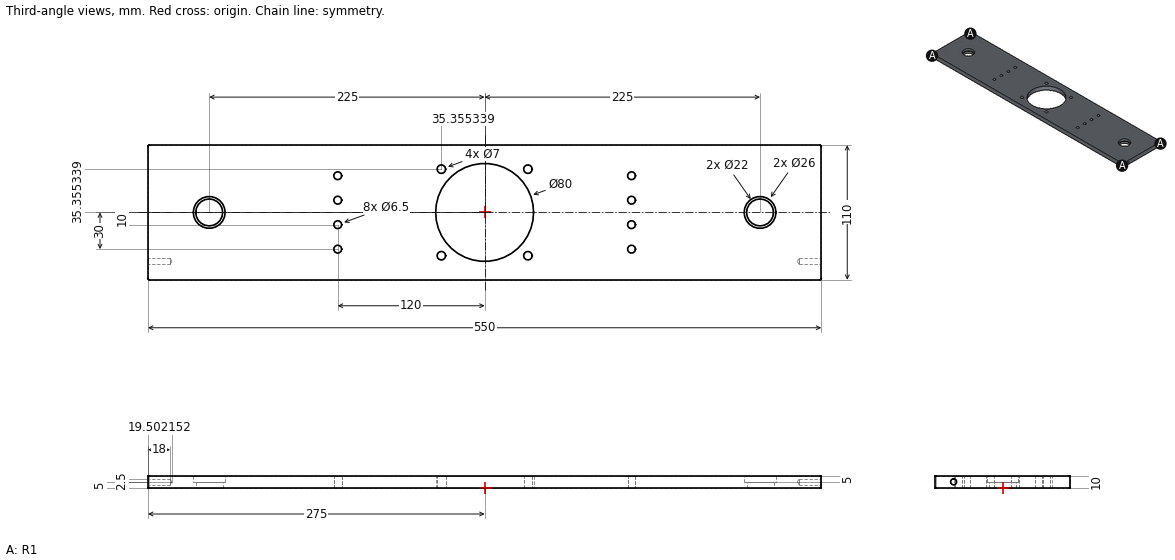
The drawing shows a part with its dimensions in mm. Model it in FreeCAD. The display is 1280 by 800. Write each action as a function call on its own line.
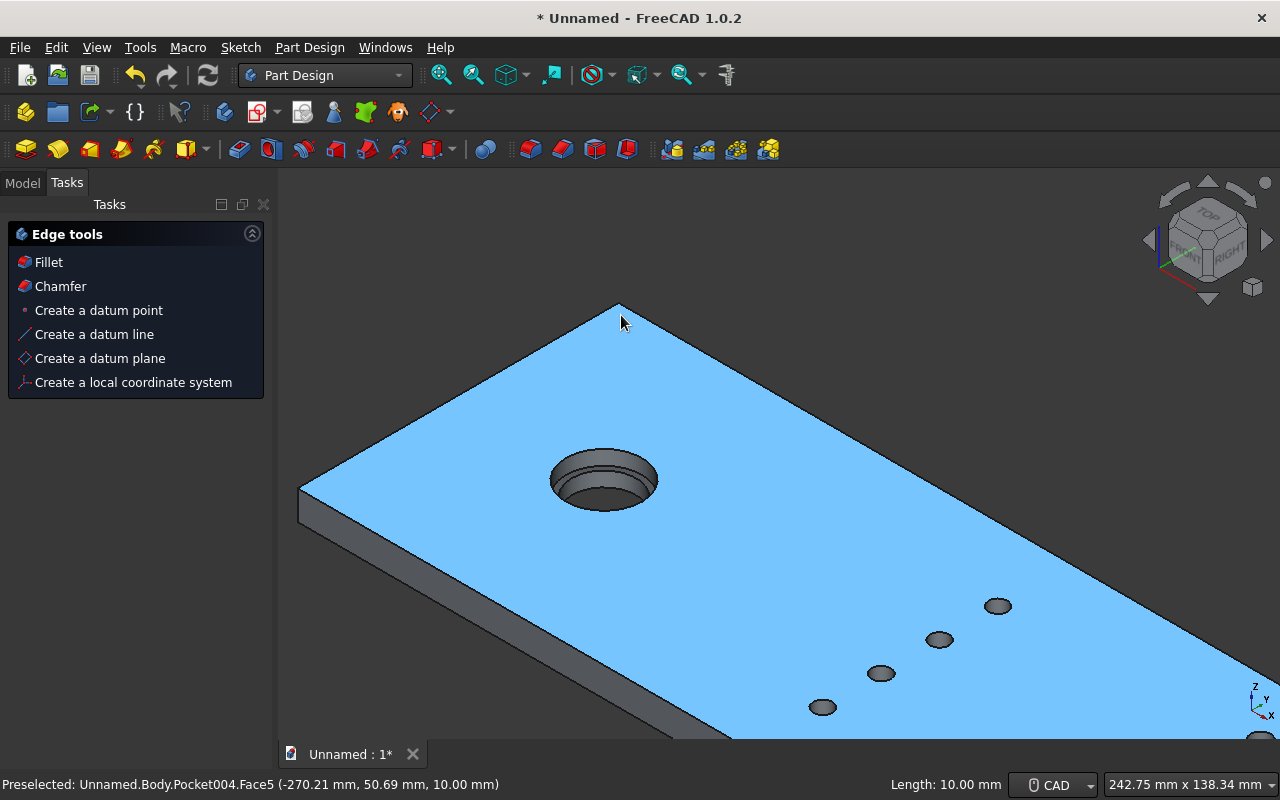
key(v)
key(f)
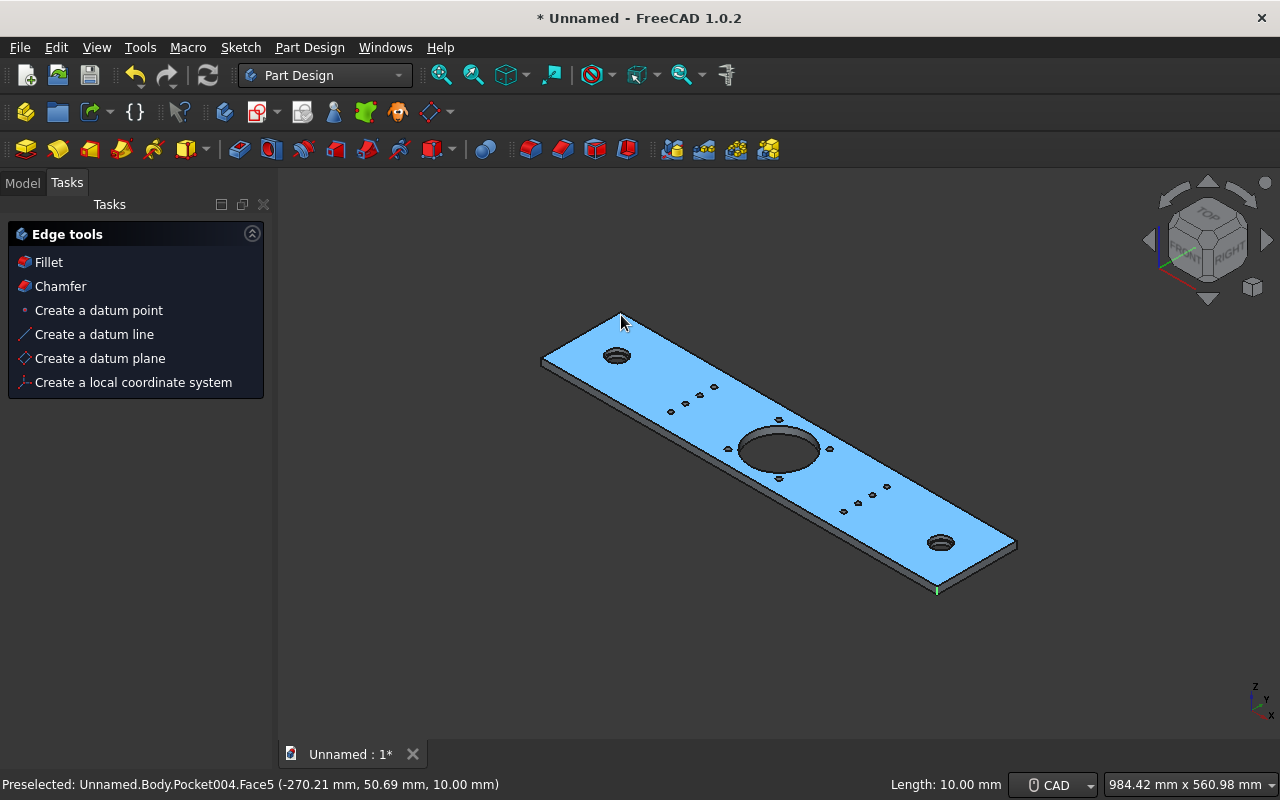
key(2)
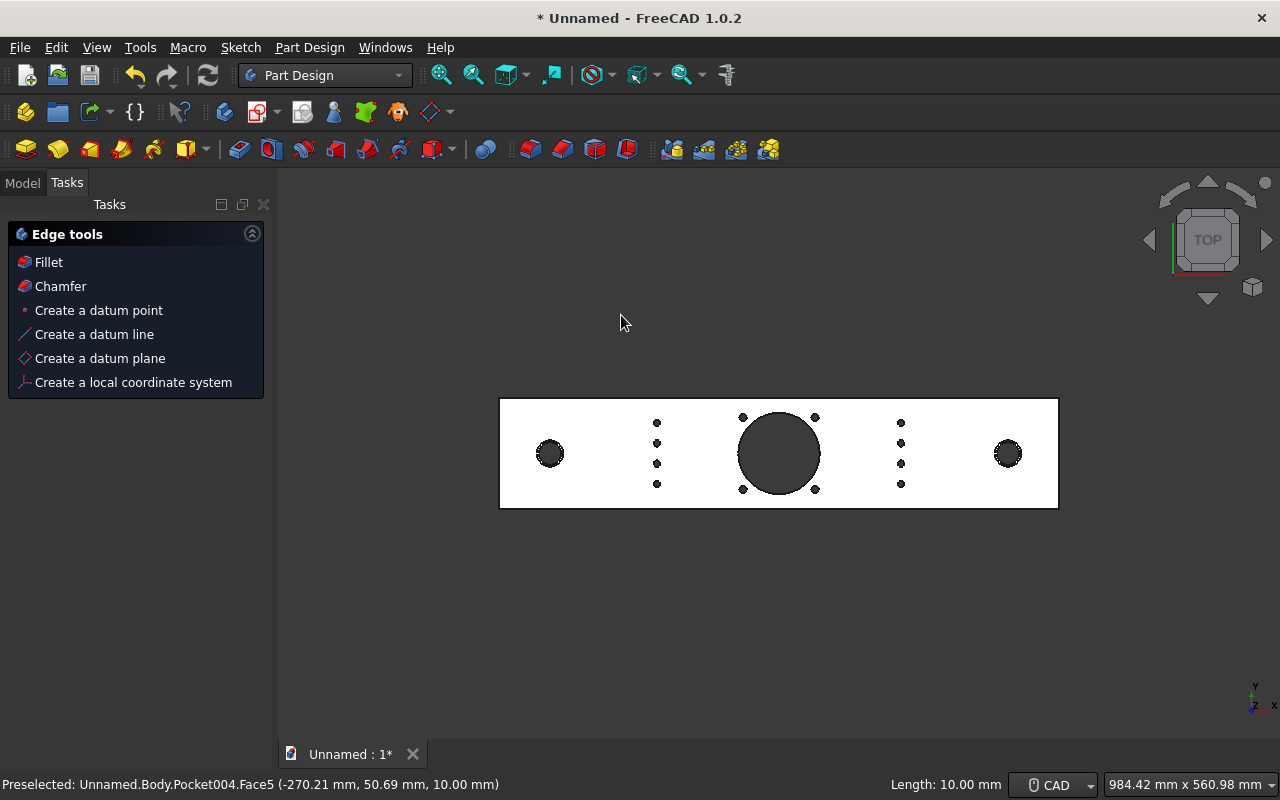
scroll(499, 397, up, 7)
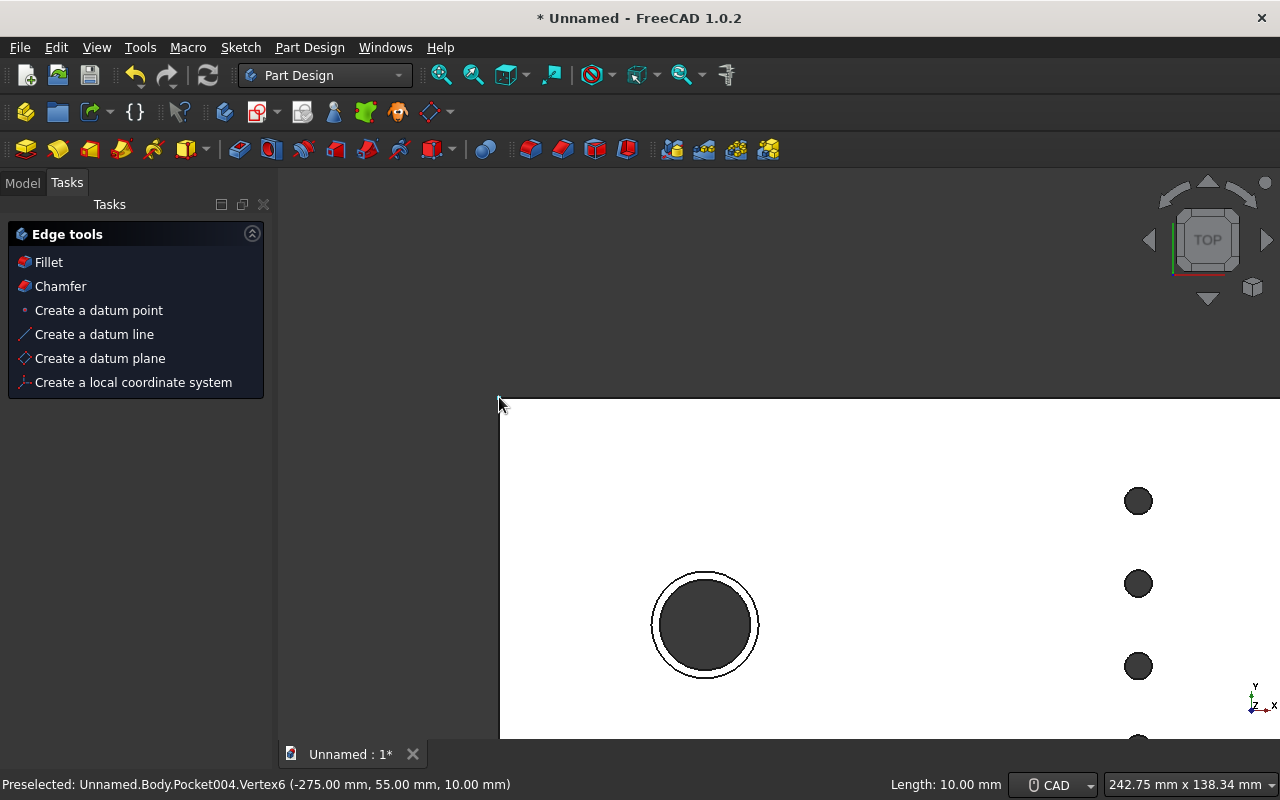
key(v)
key(f)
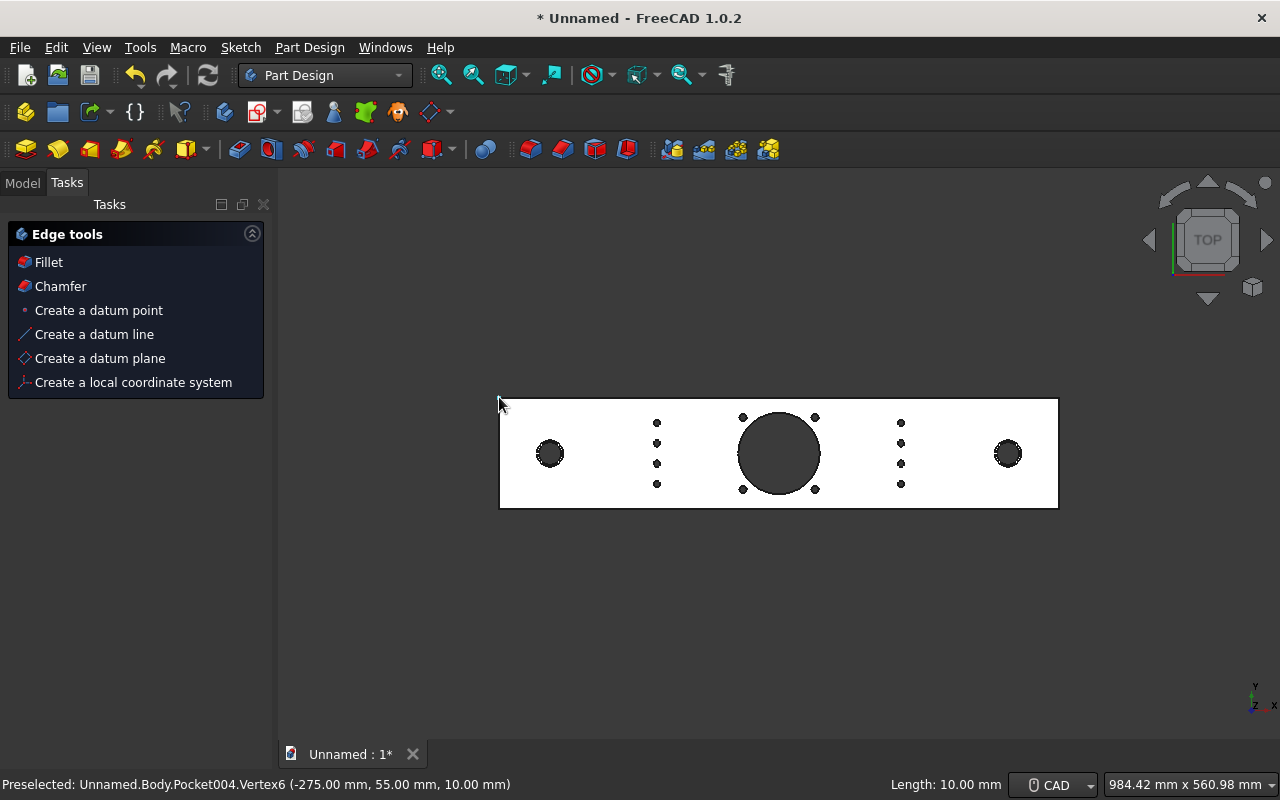
key(1)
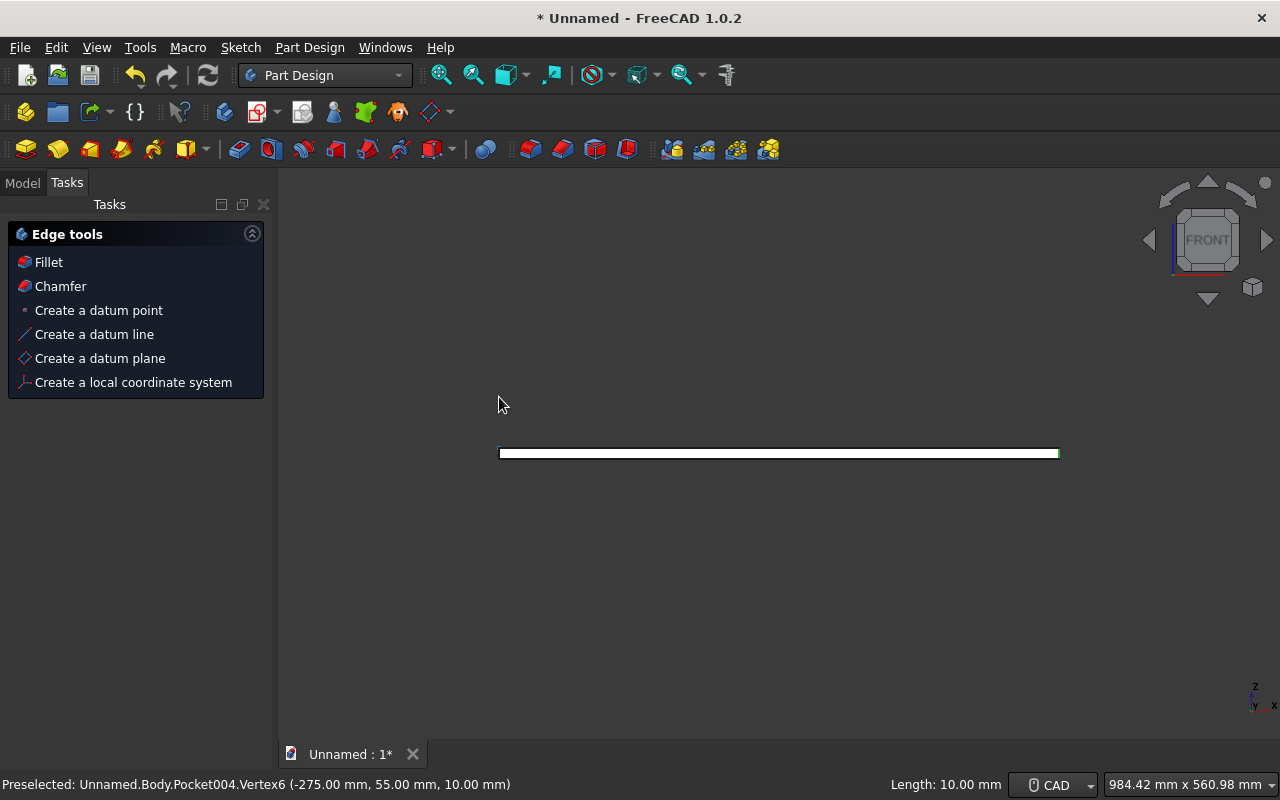
scroll(499, 452, up, 7)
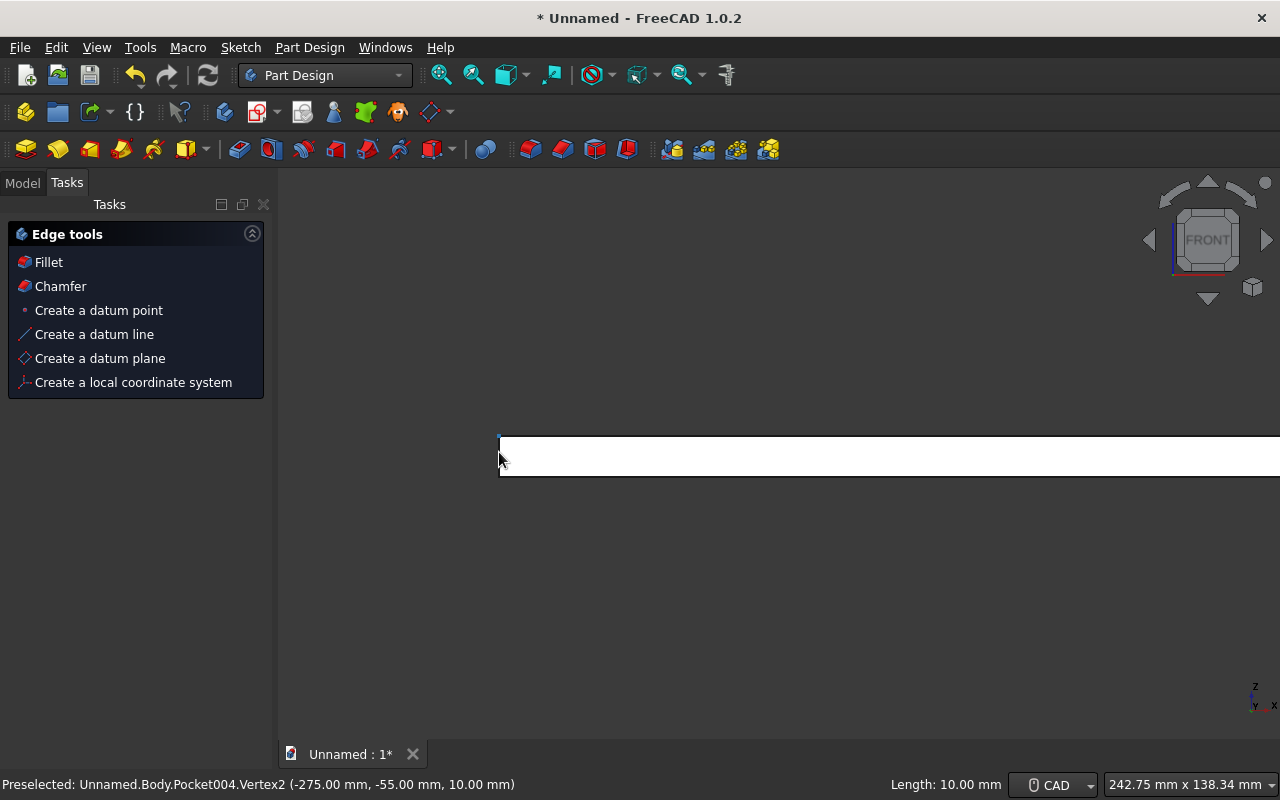
click(499, 456, ctrl)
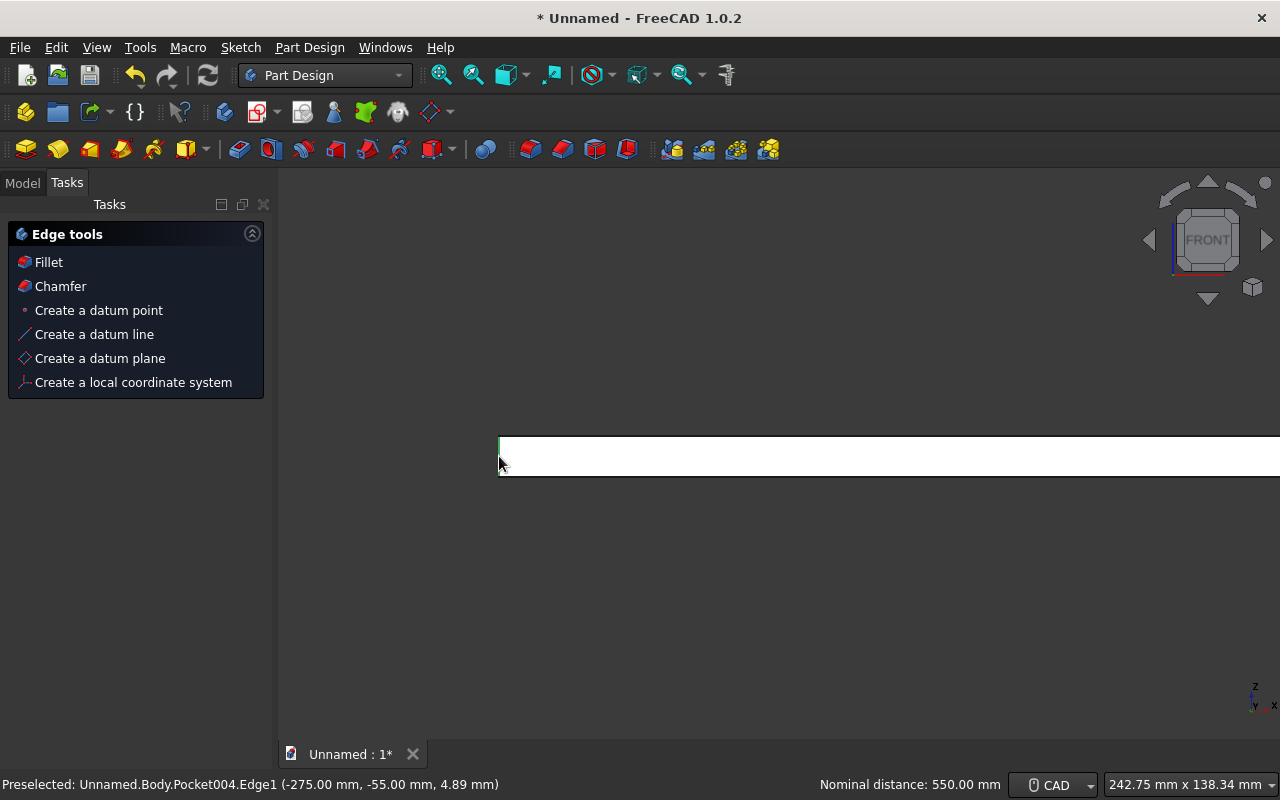
key(v)
key(f)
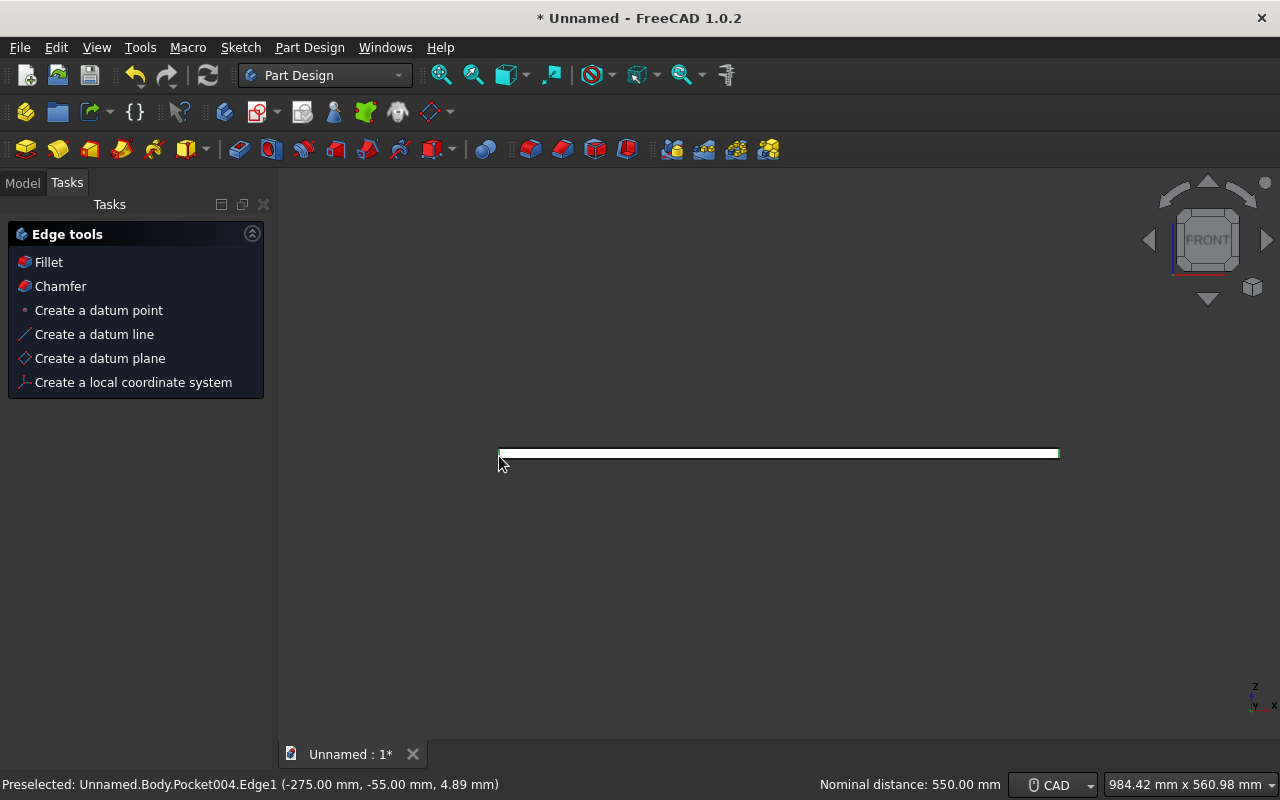
key(3)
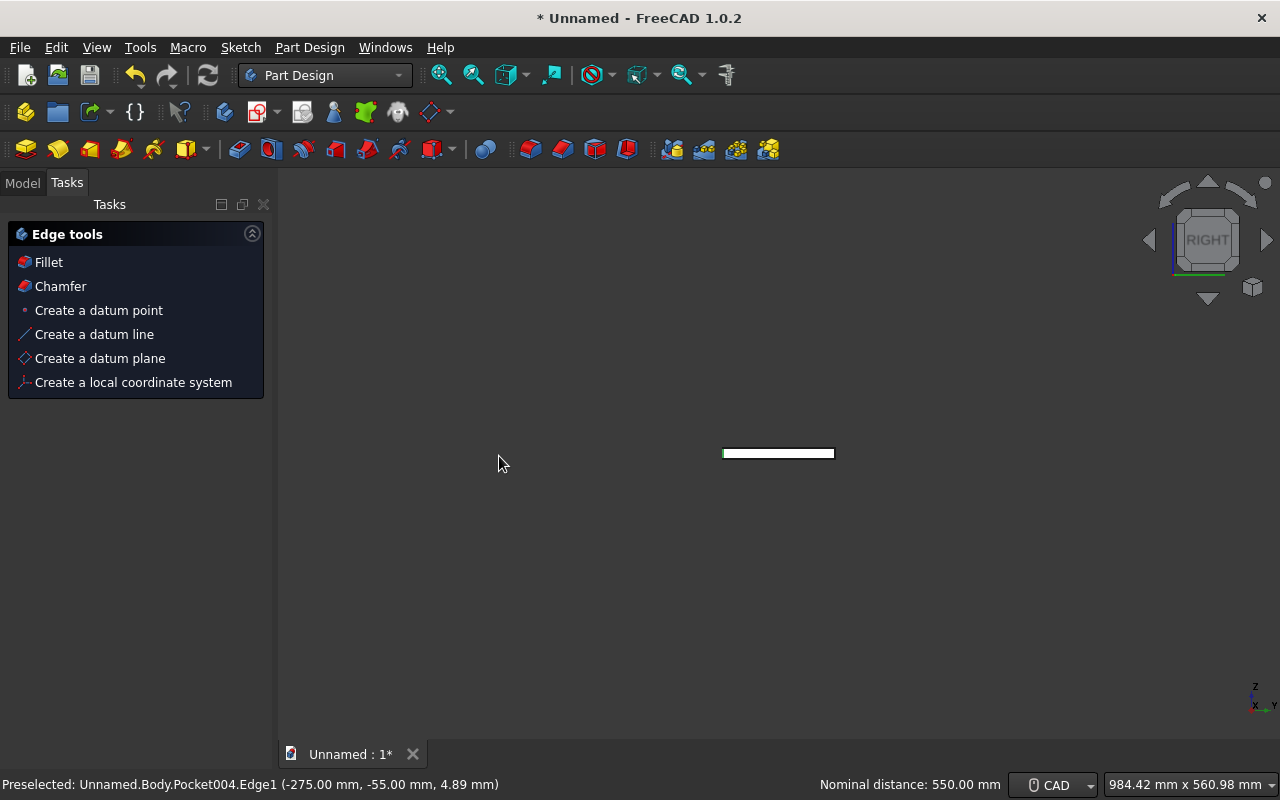
click(442, 76)